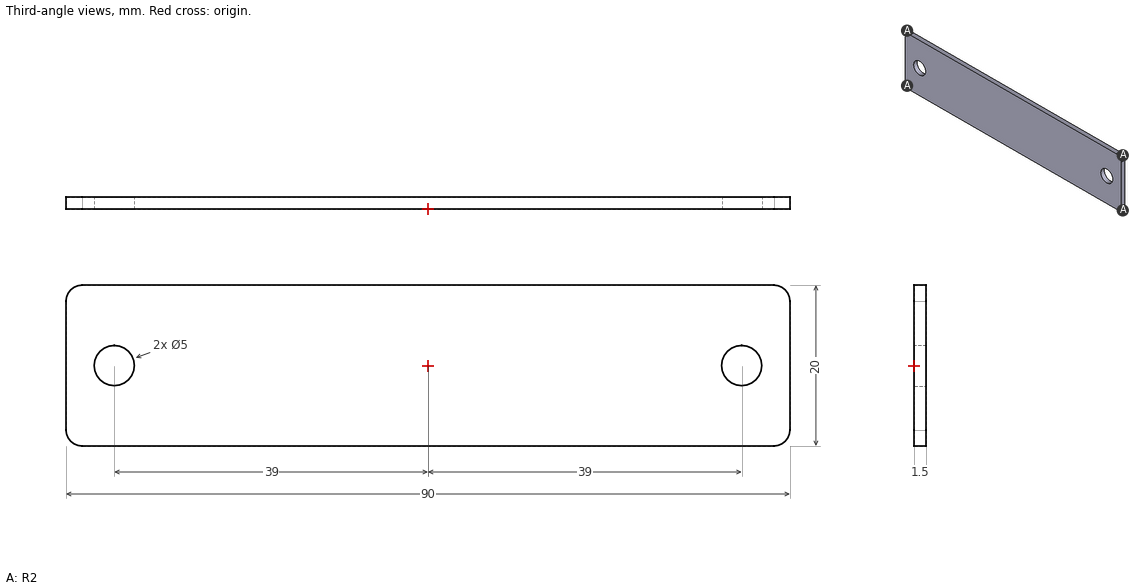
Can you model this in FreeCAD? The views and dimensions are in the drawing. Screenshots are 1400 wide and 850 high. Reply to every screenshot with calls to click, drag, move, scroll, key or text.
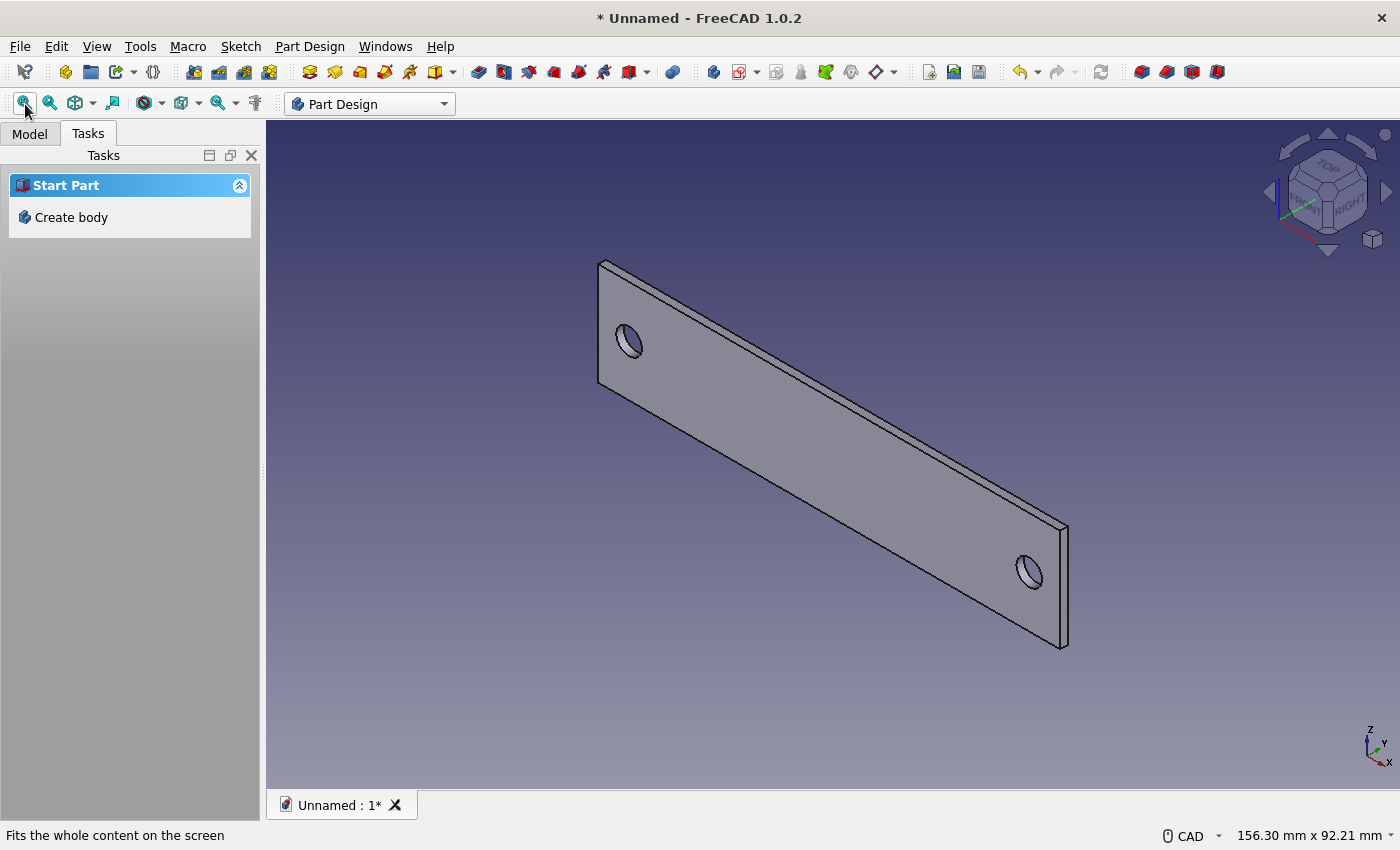
scroll(1064, 528, up, 7)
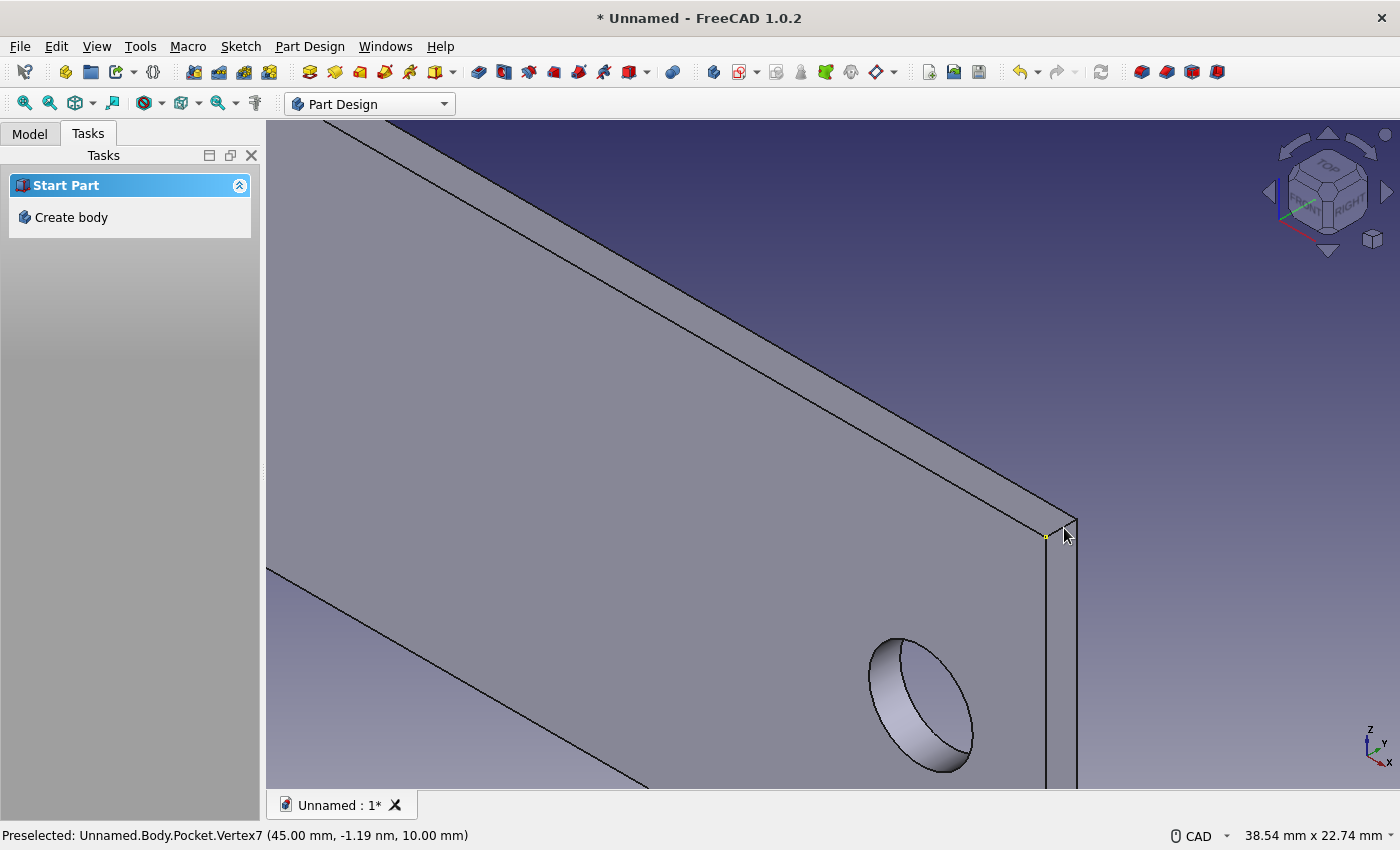
click(1061, 527)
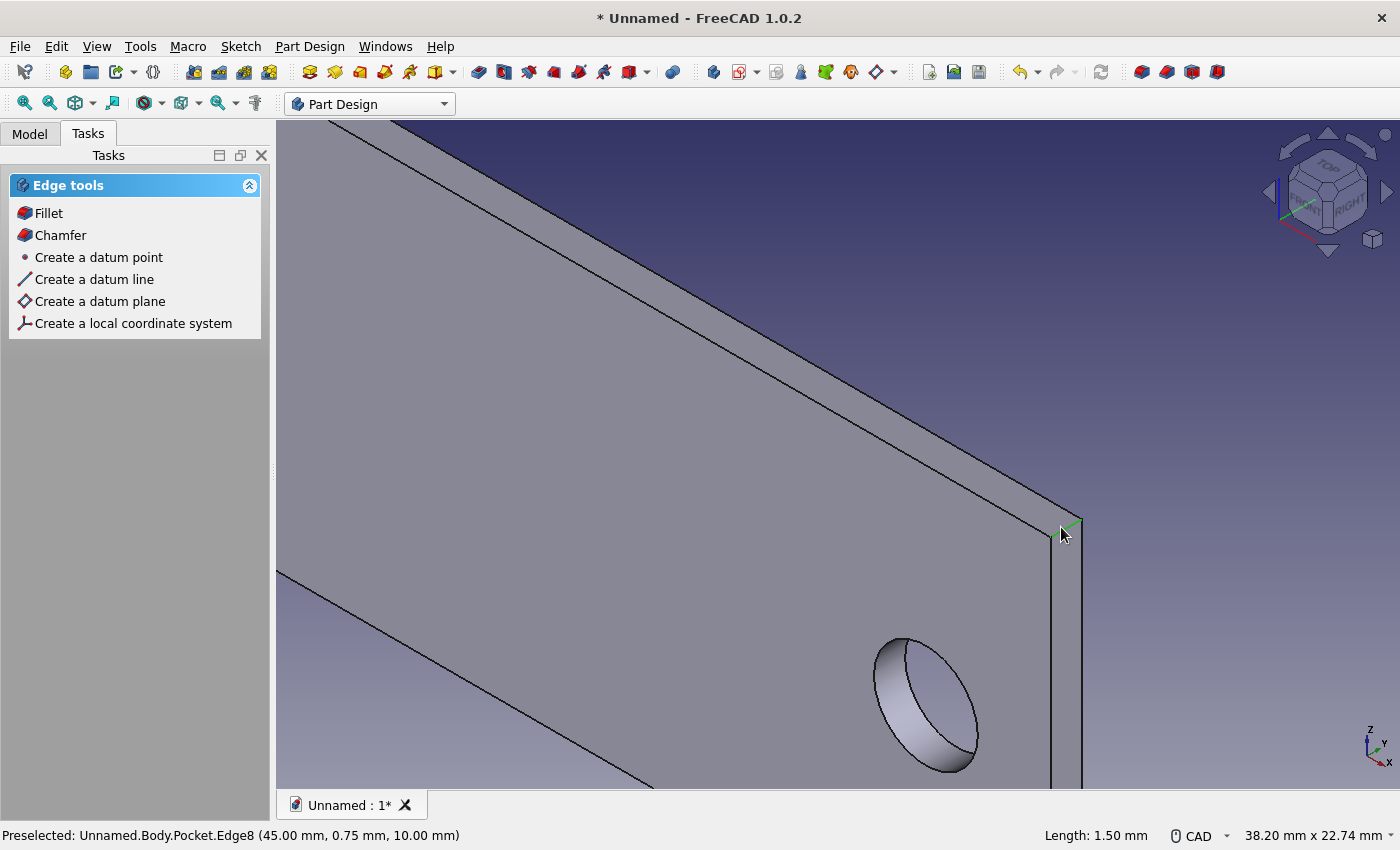
click(25, 104)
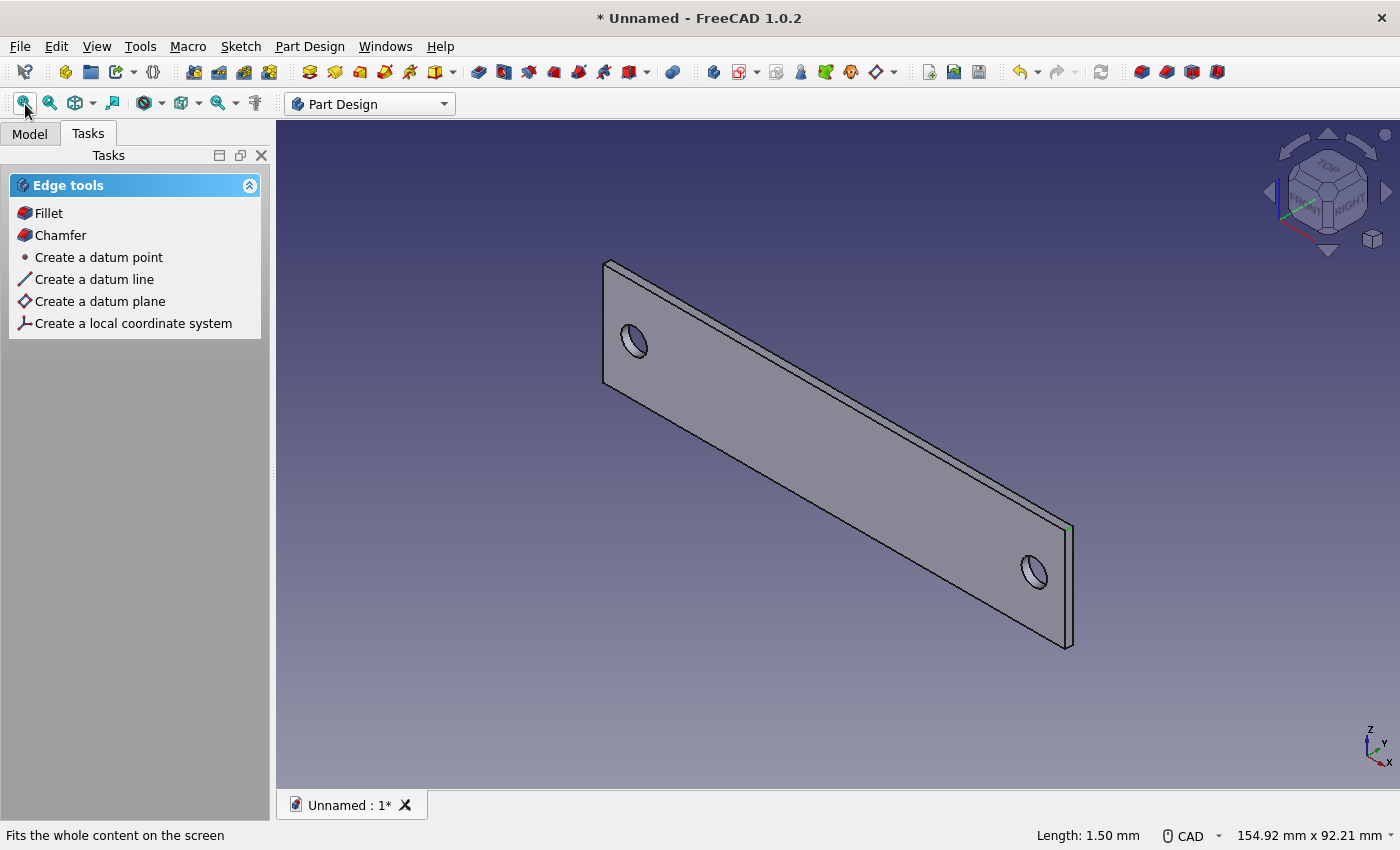
key(2)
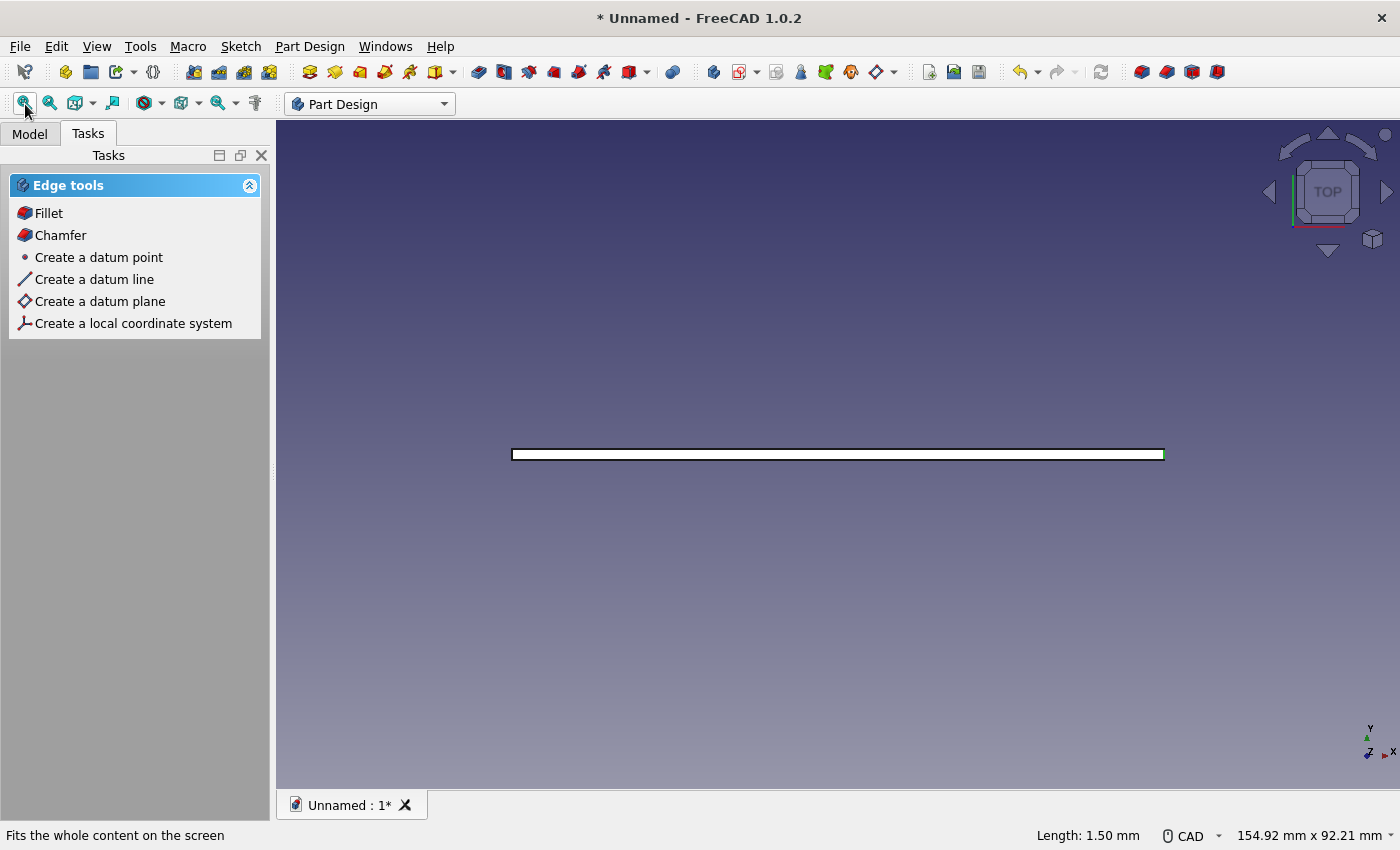
click(512, 455, ctrl)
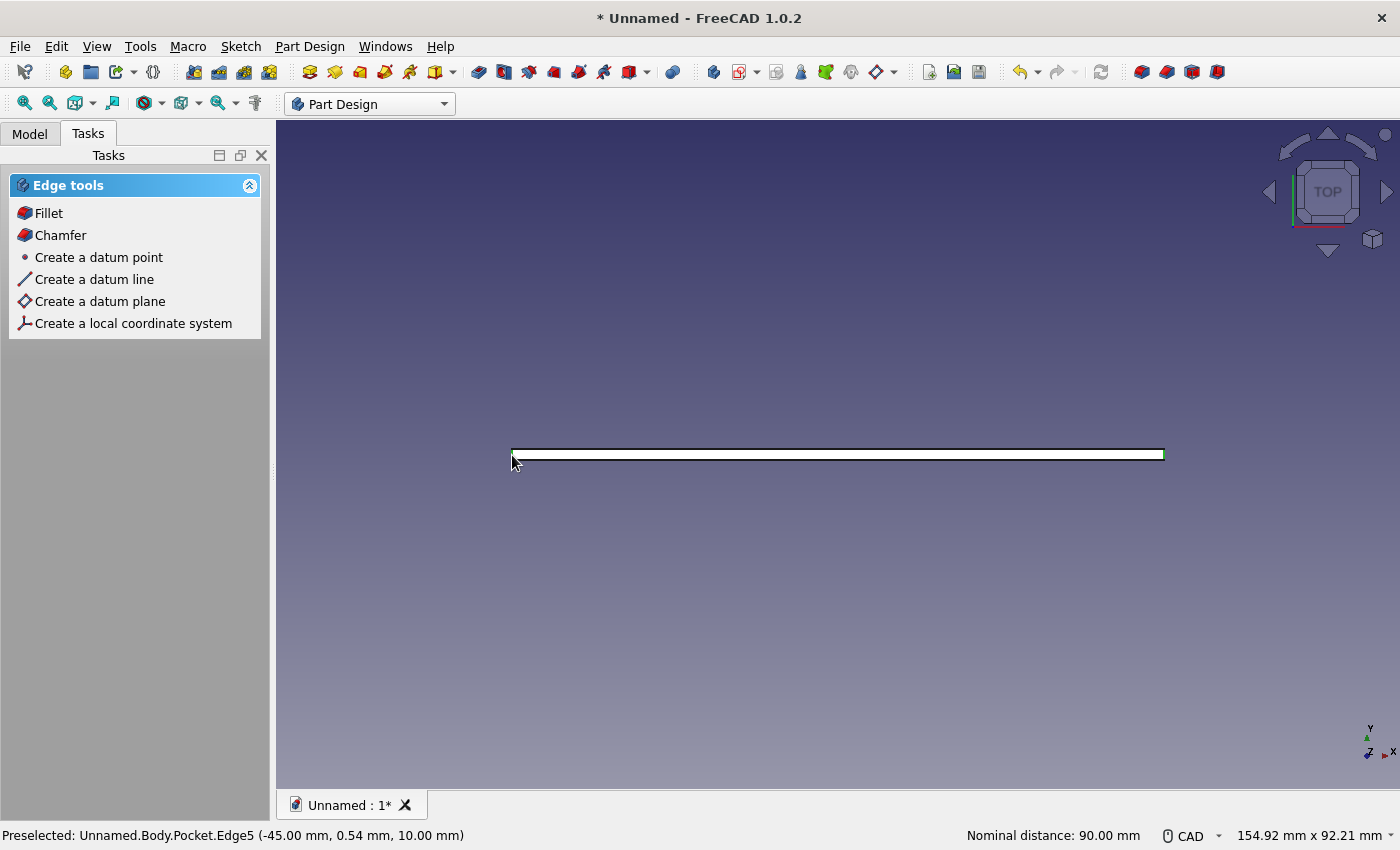
scroll(512, 453, up, 7)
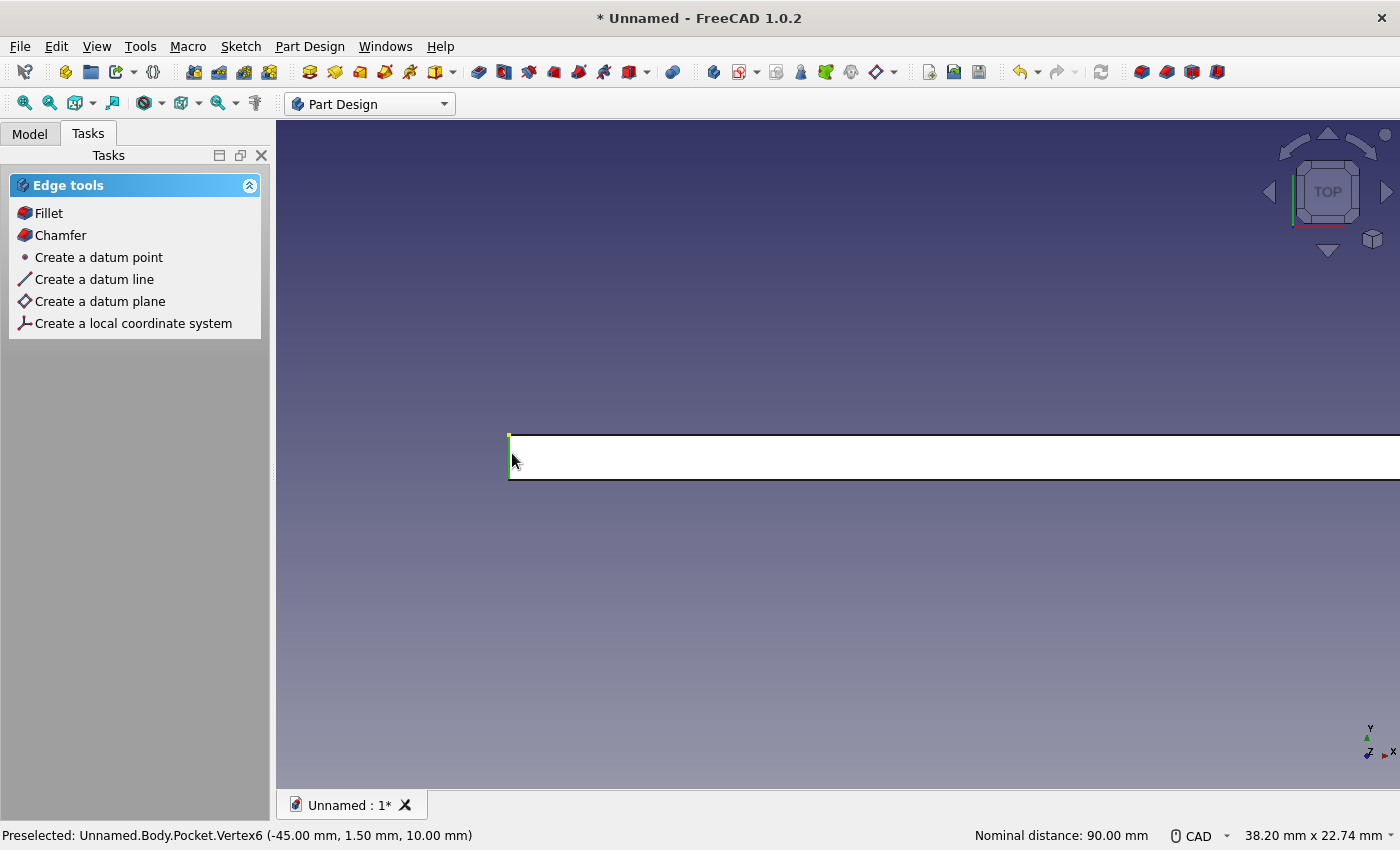
click(25, 104)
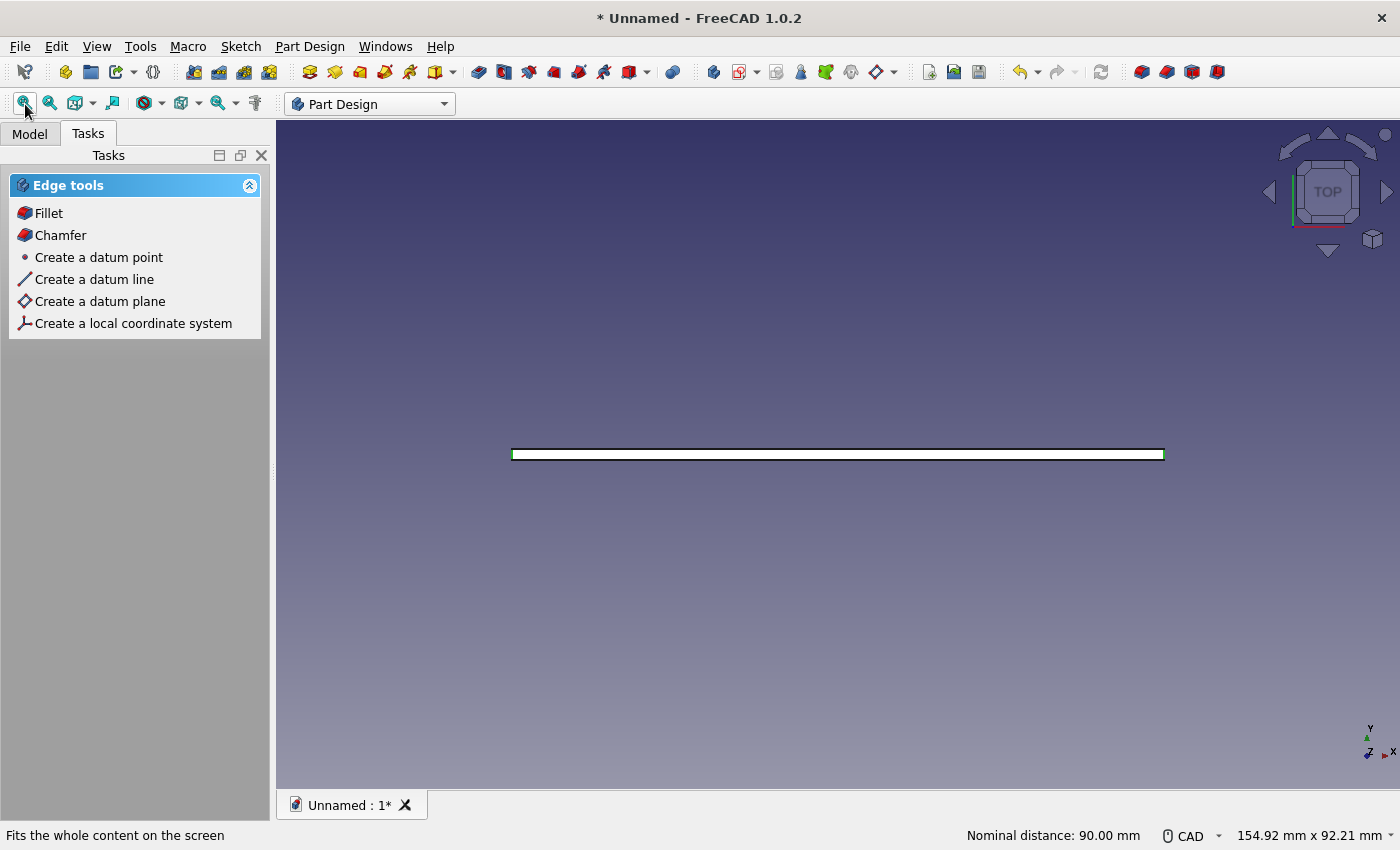
key(1)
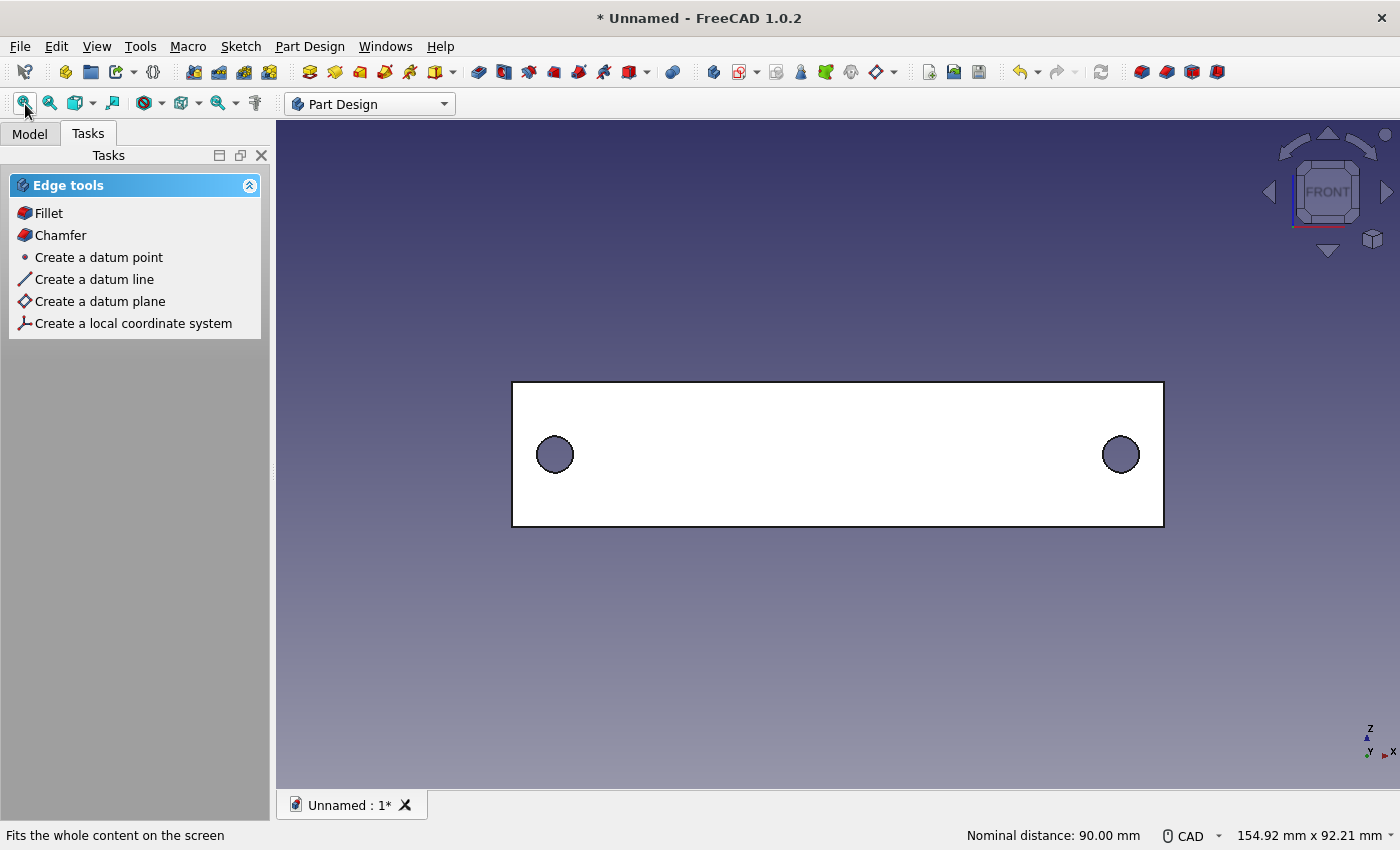
scroll(512, 526, up, 7)